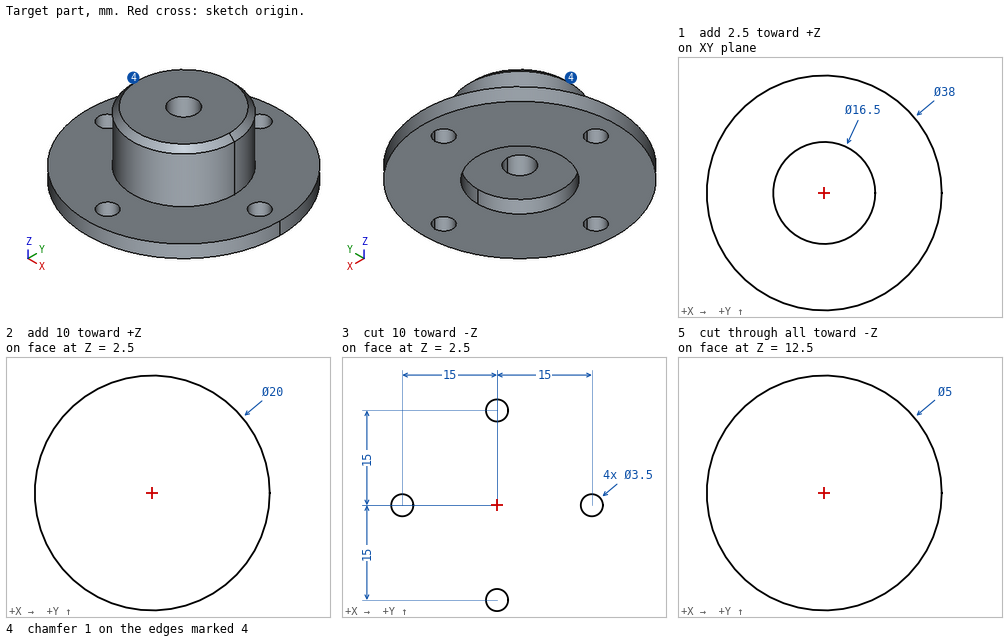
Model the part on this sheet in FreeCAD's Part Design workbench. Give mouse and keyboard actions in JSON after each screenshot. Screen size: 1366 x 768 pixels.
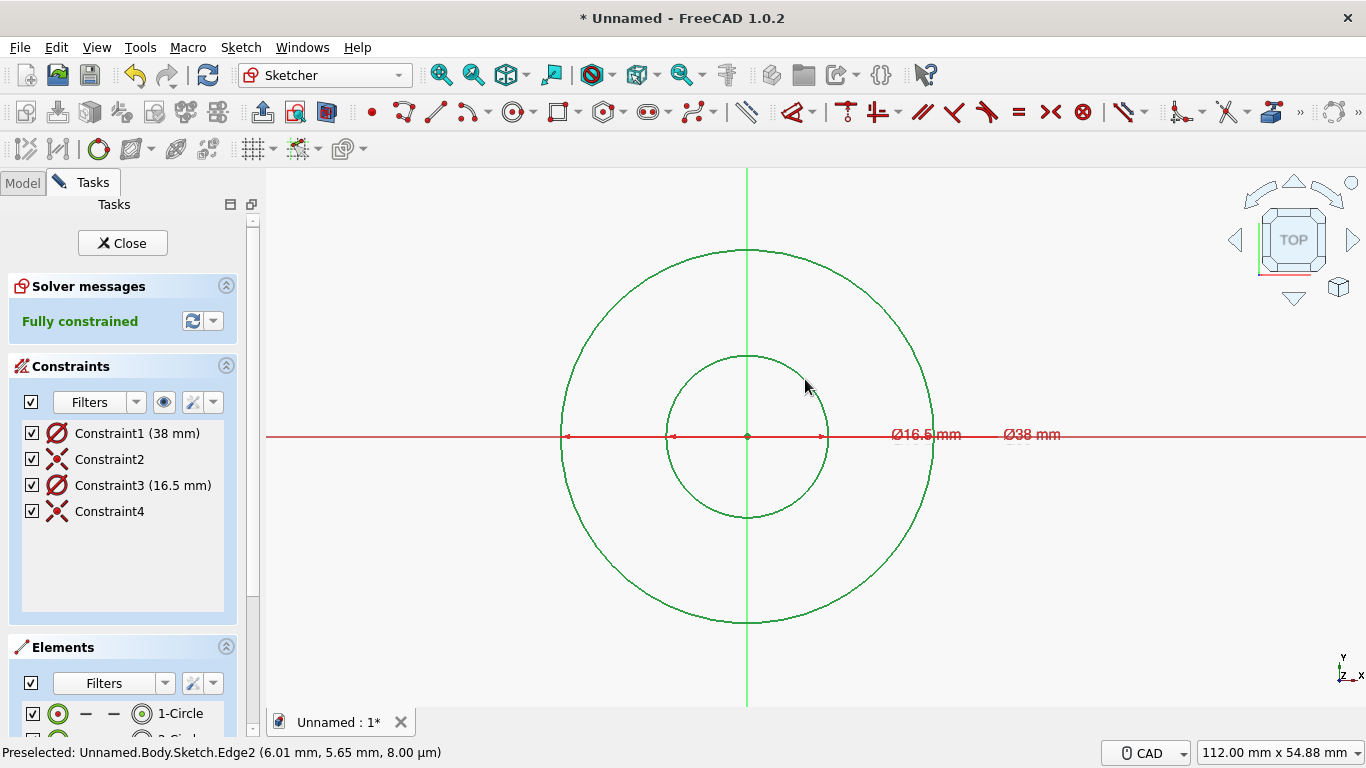
{"action": "left_click", "coordinate": [123, 243]}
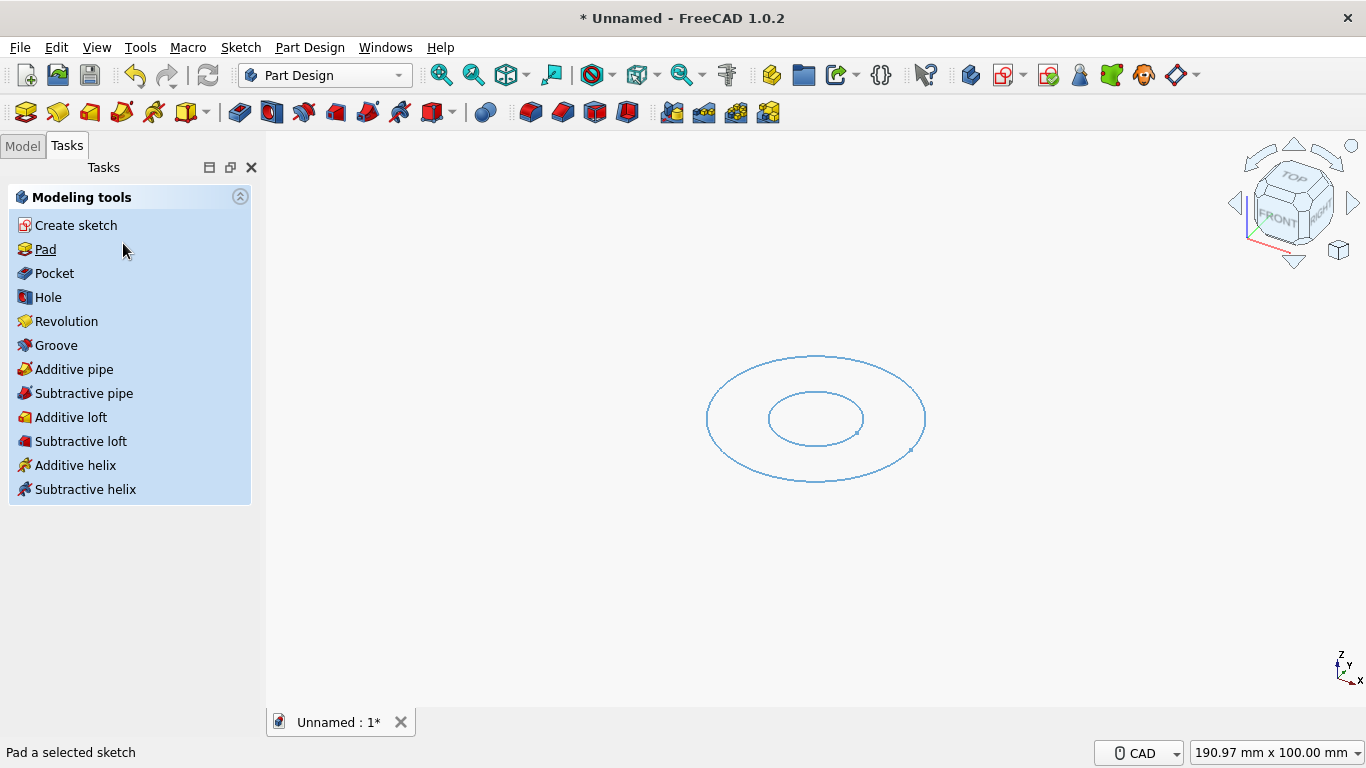
{"action": "left_click", "coordinate": [26, 112]}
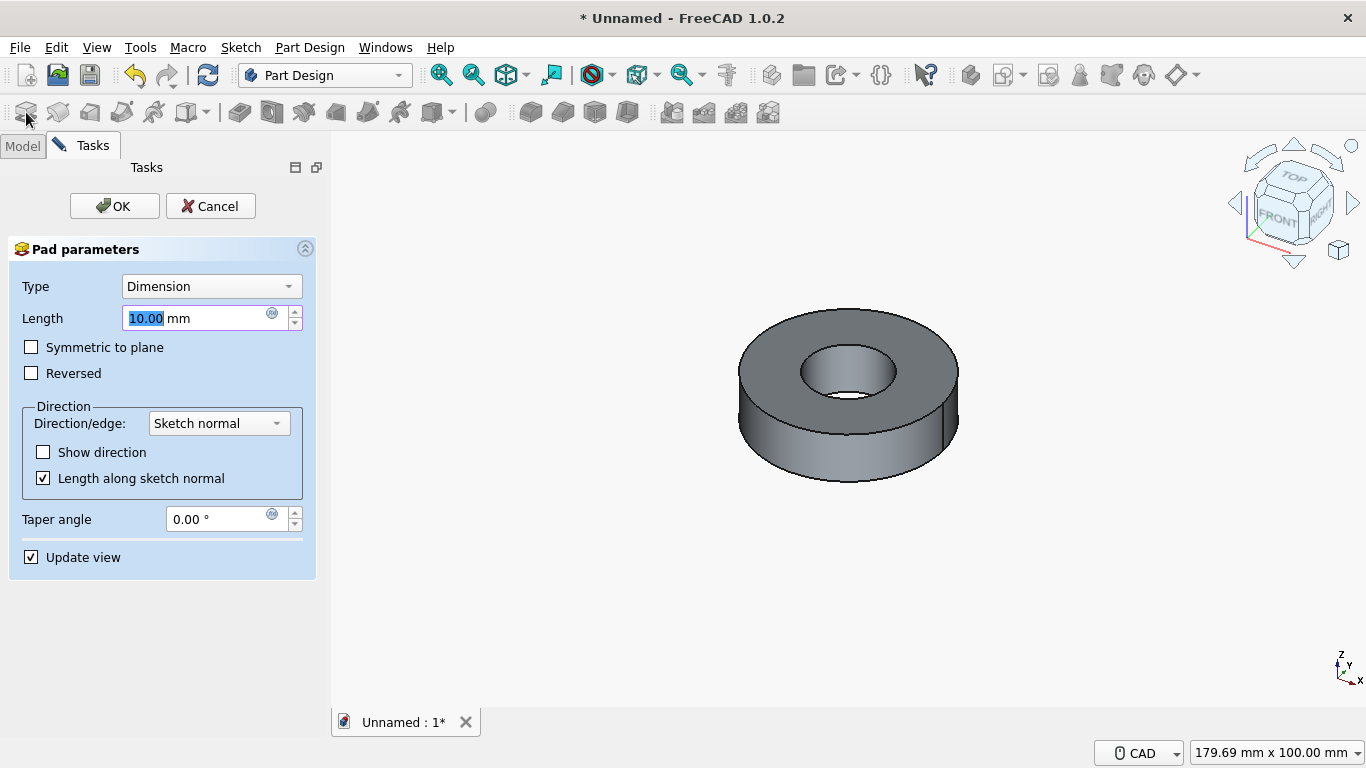
{"action": "type", "text": "2.5"}
{"action": "key", "text": "Tab"}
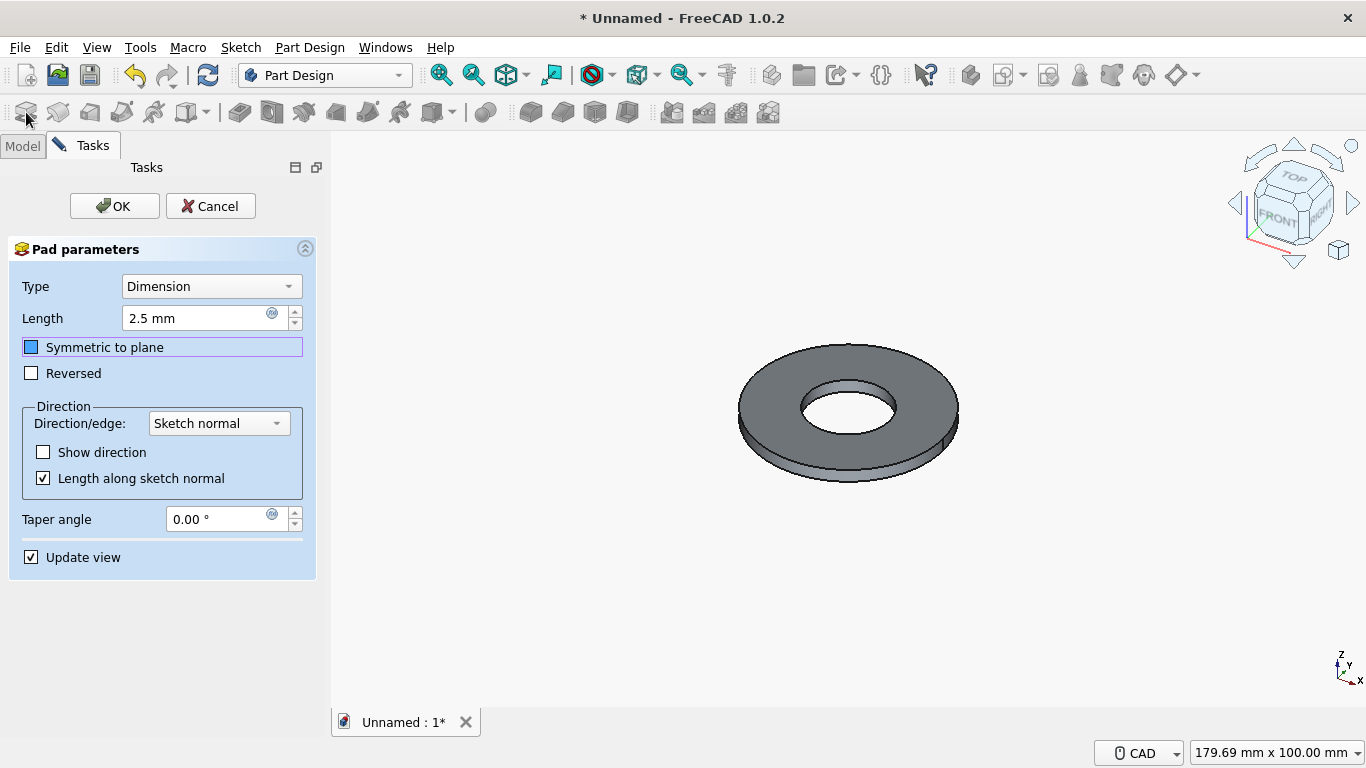
{"action": "left_click", "coordinate": [115, 206]}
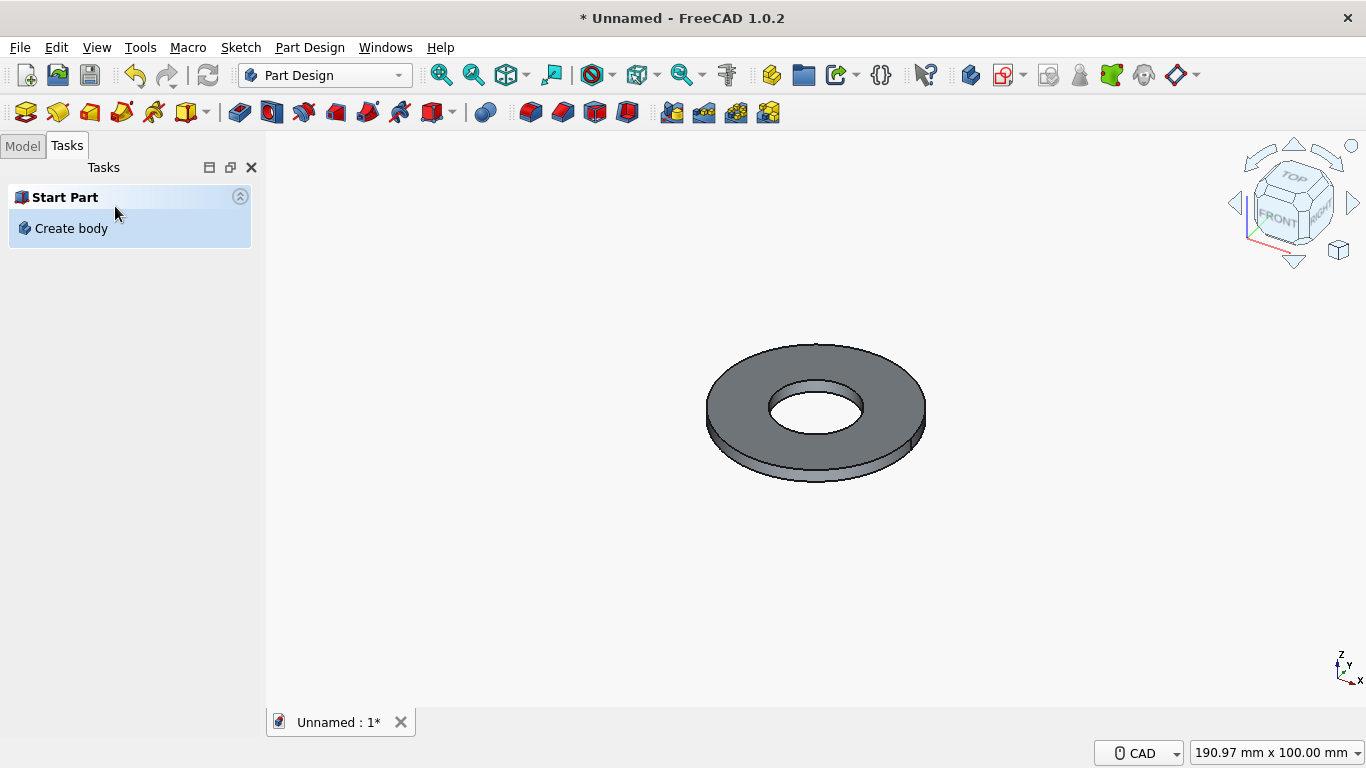
{"action": "key", "text": "v f"}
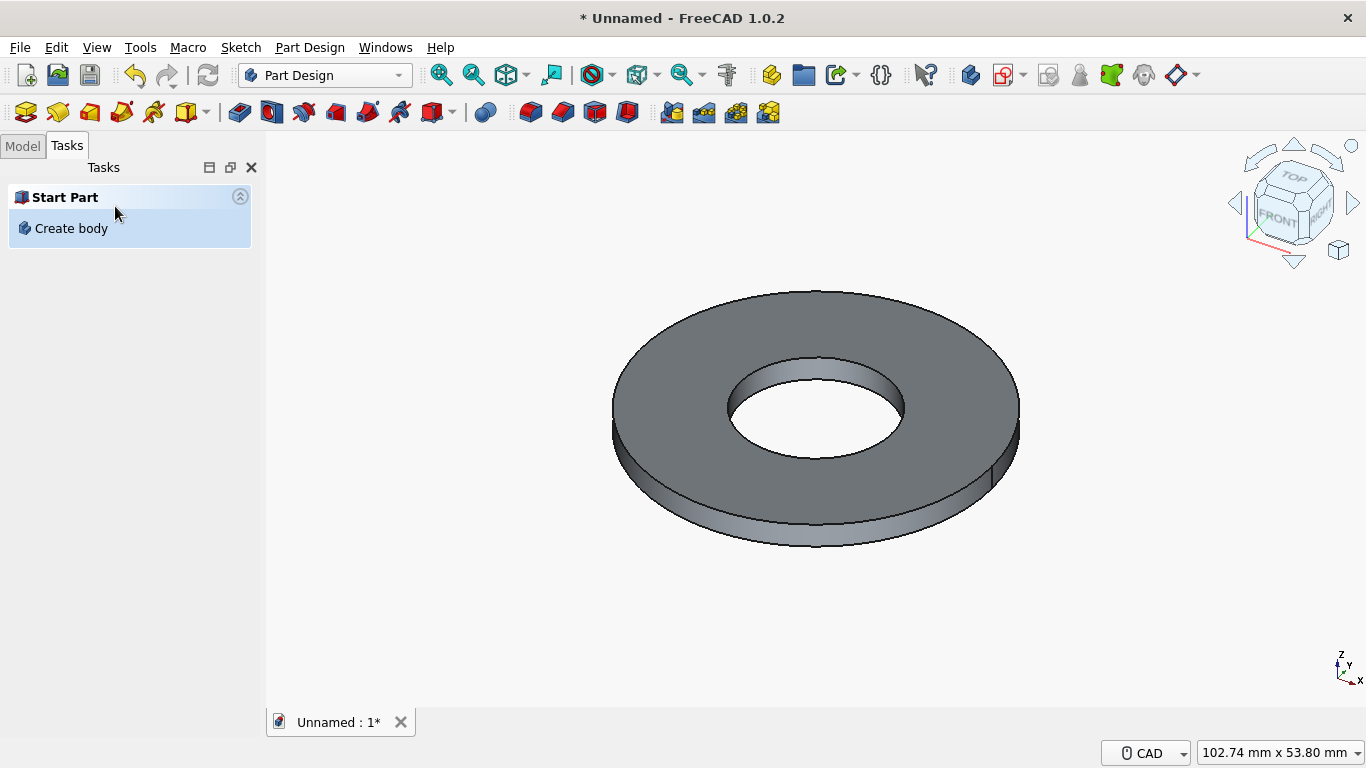
{"action": "left_click", "coordinate": [824, 333]}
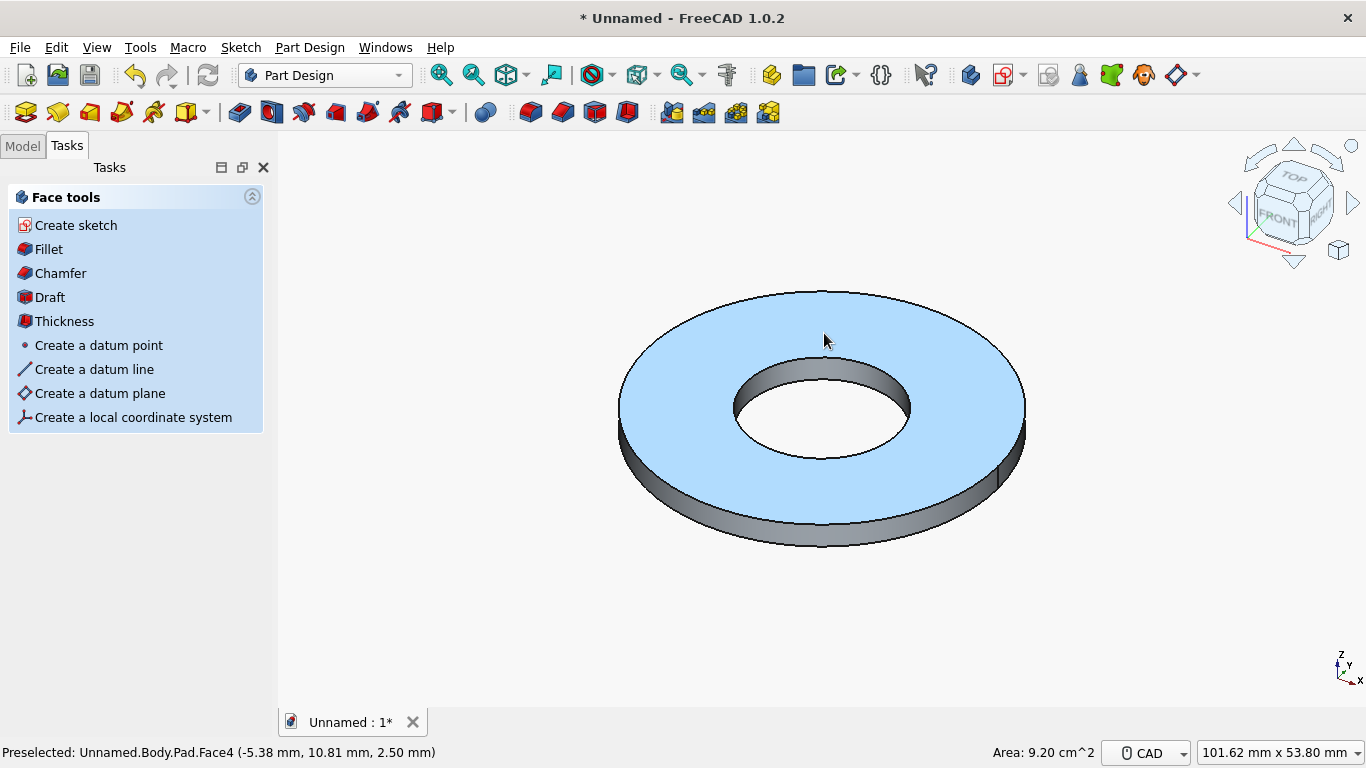
{"action": "left_click", "coordinate": [1004, 76]}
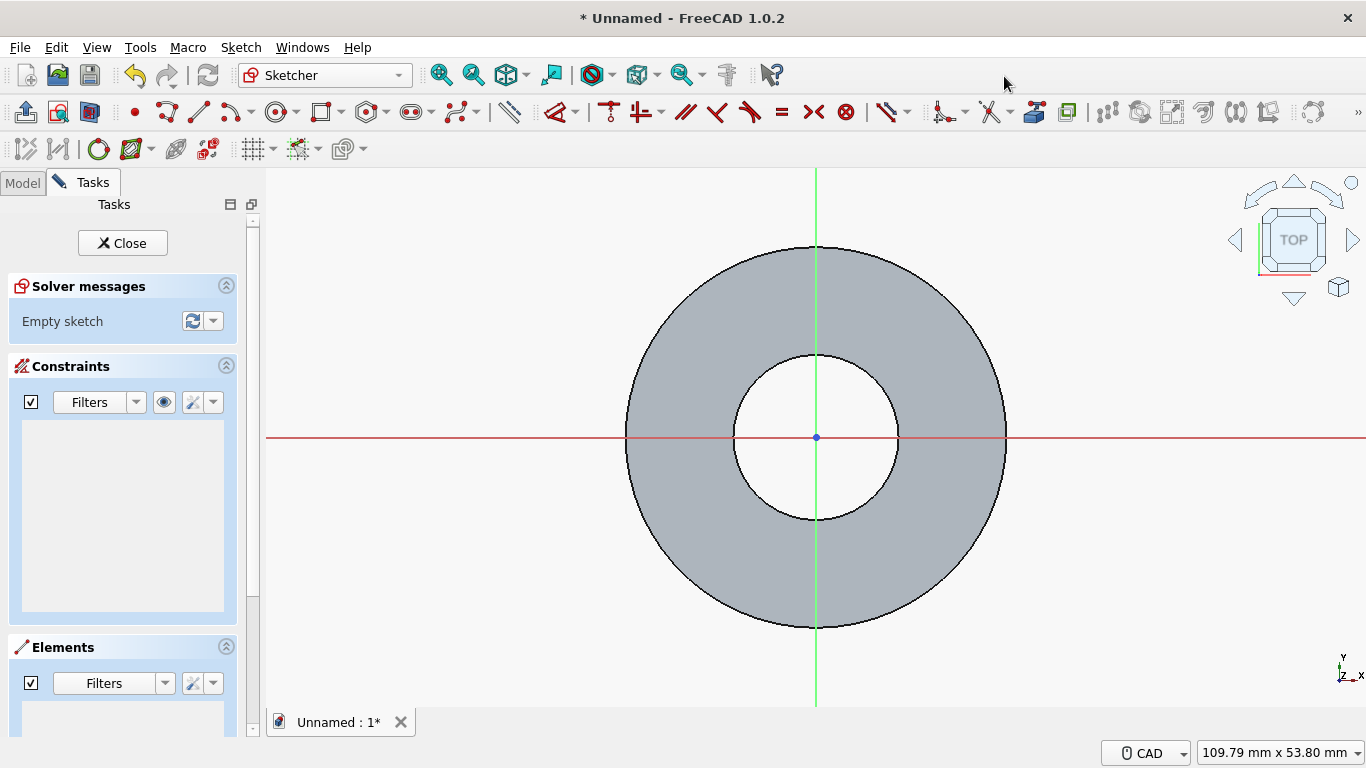
{"action": "scroll", "coordinate": [899, 438], "scroll_direction": "up", "scroll_amount": 3}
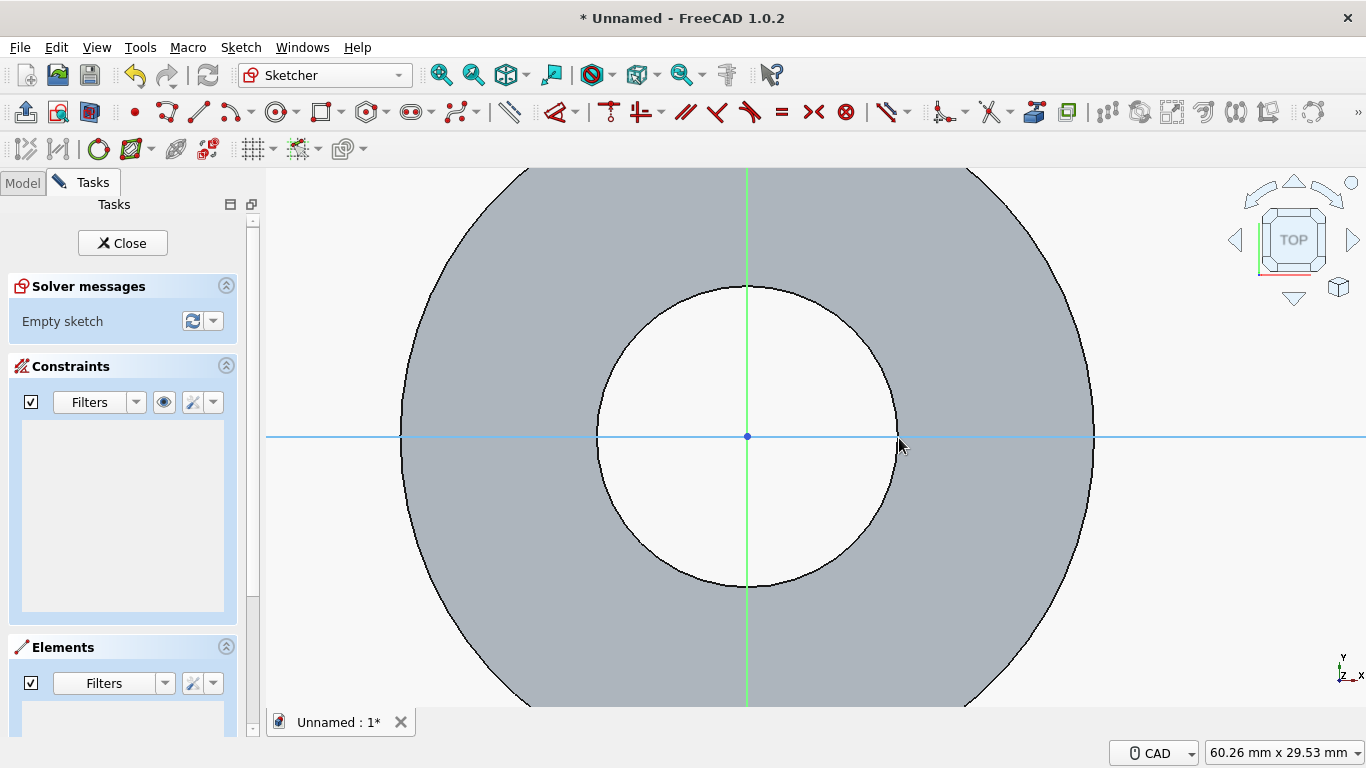
{"action": "key", "text": "g c"}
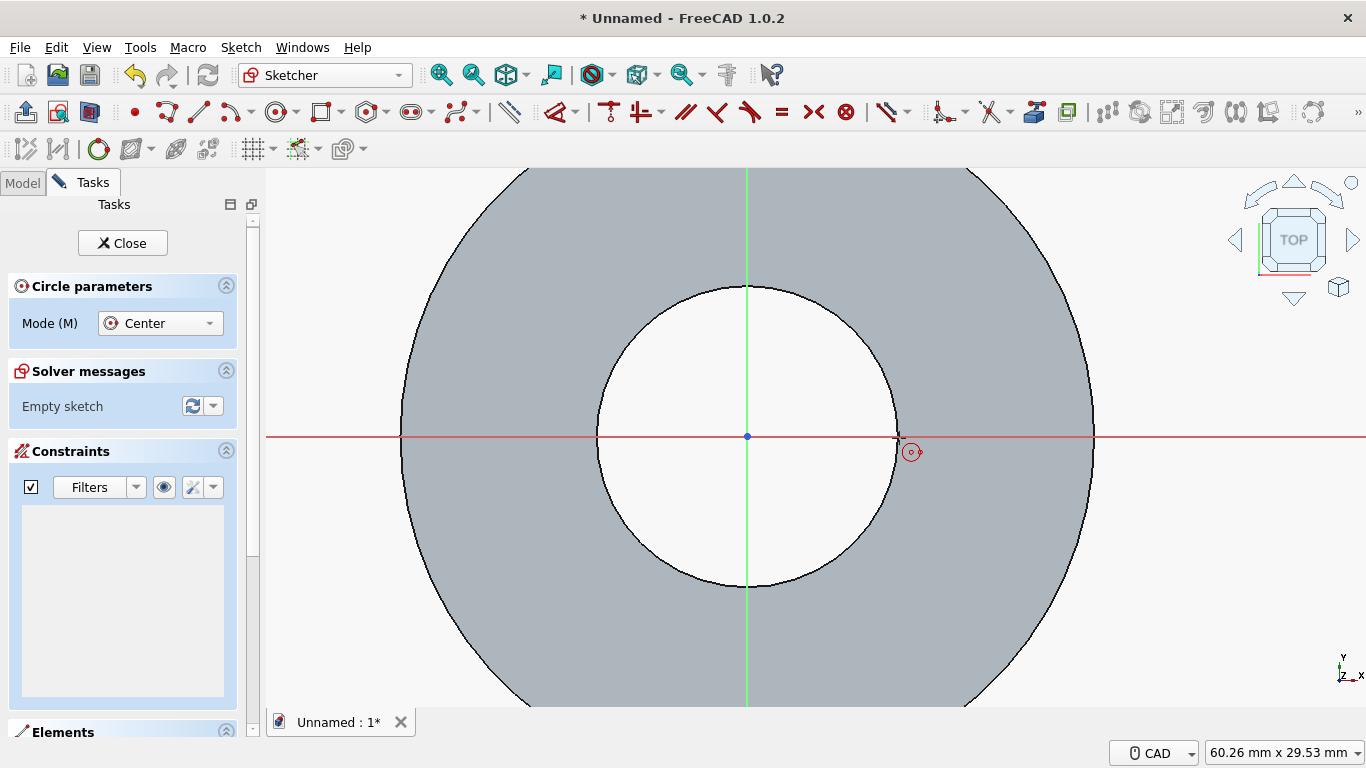
{"action": "left_click", "coordinate": [747, 437]}
{"action": "mouse_move", "coordinate": [876, 308]}